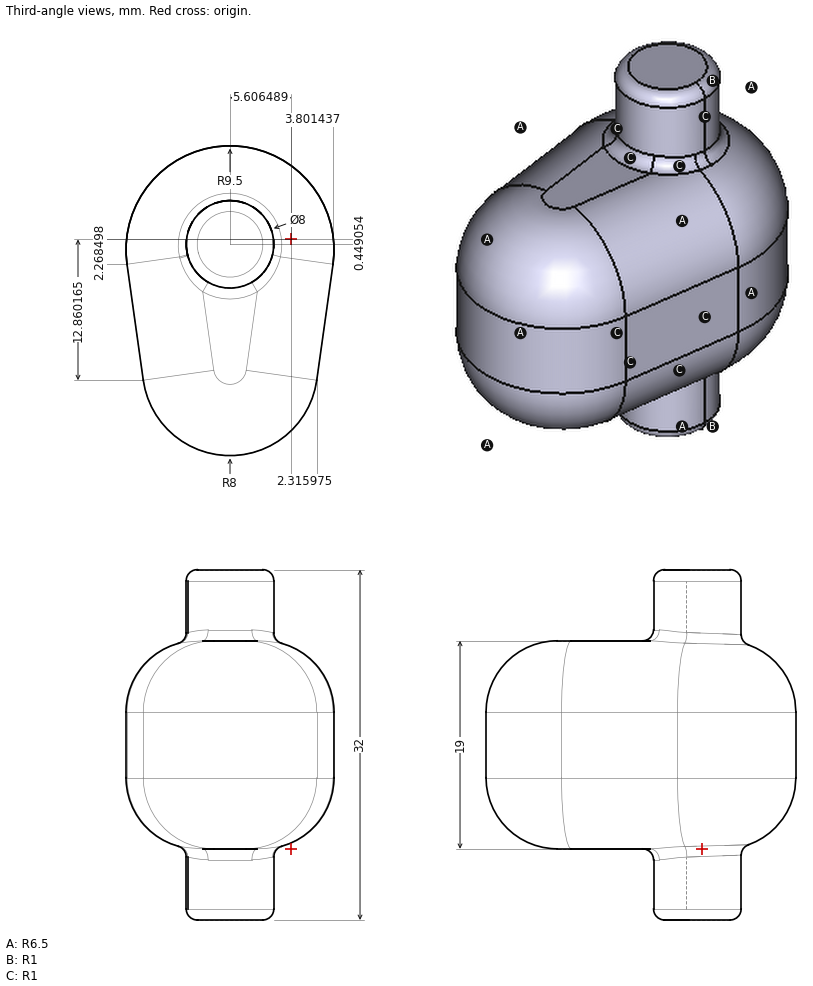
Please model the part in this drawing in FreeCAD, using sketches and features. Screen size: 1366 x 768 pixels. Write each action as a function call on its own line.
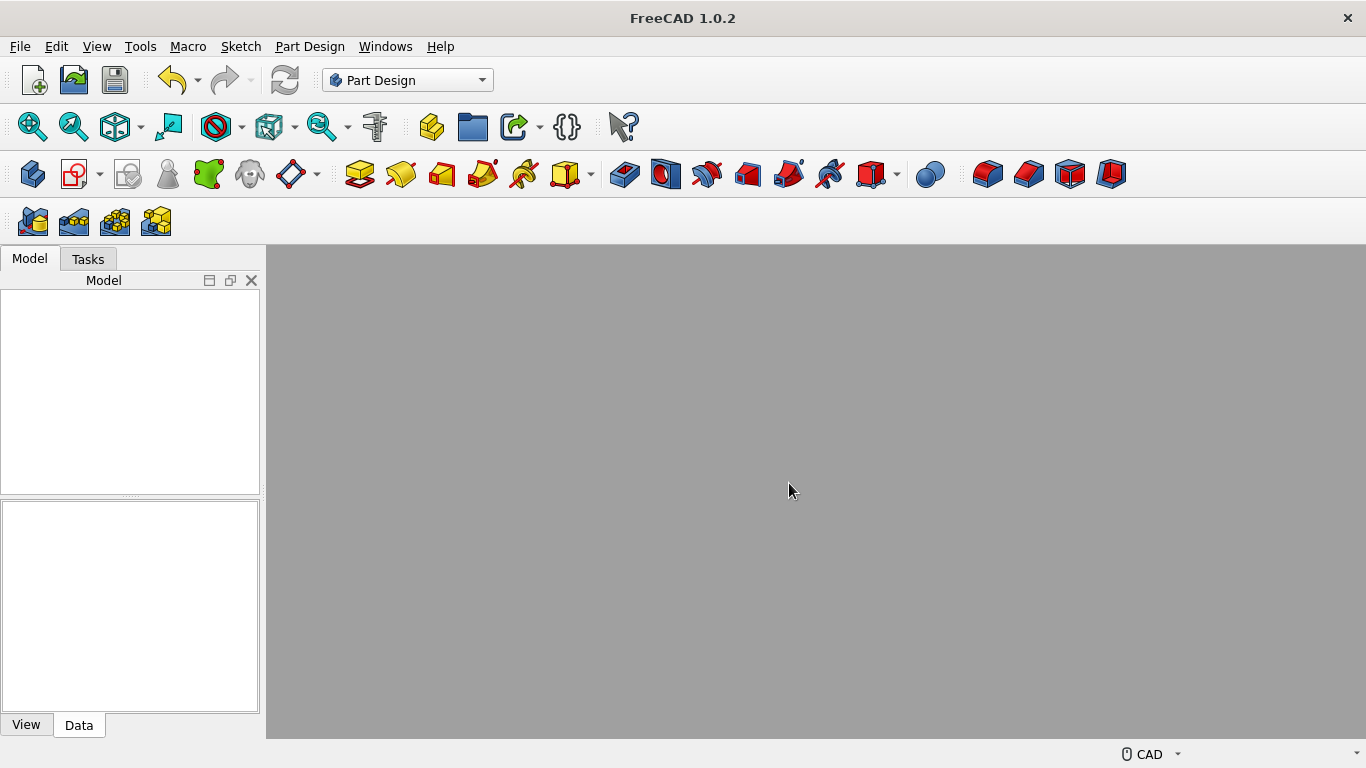
key(ctrl+n)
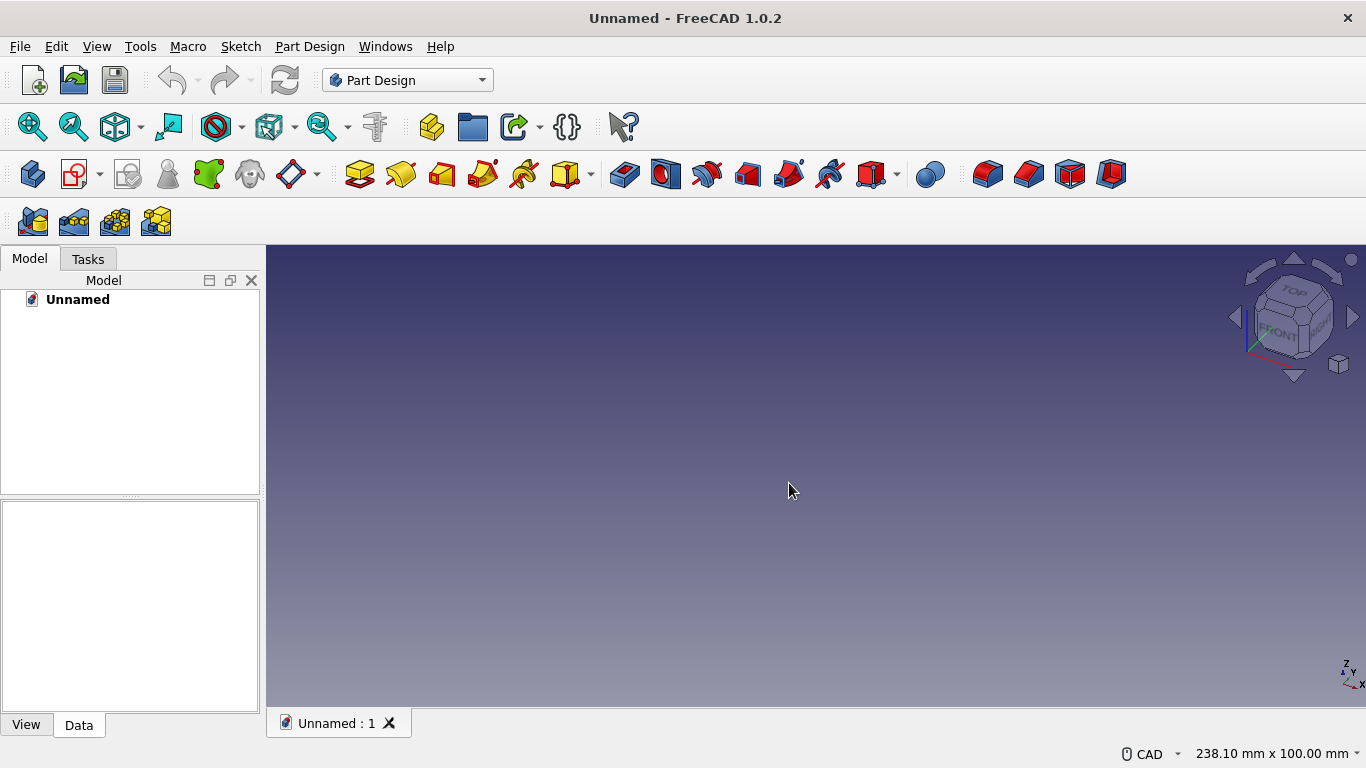
click(74, 174)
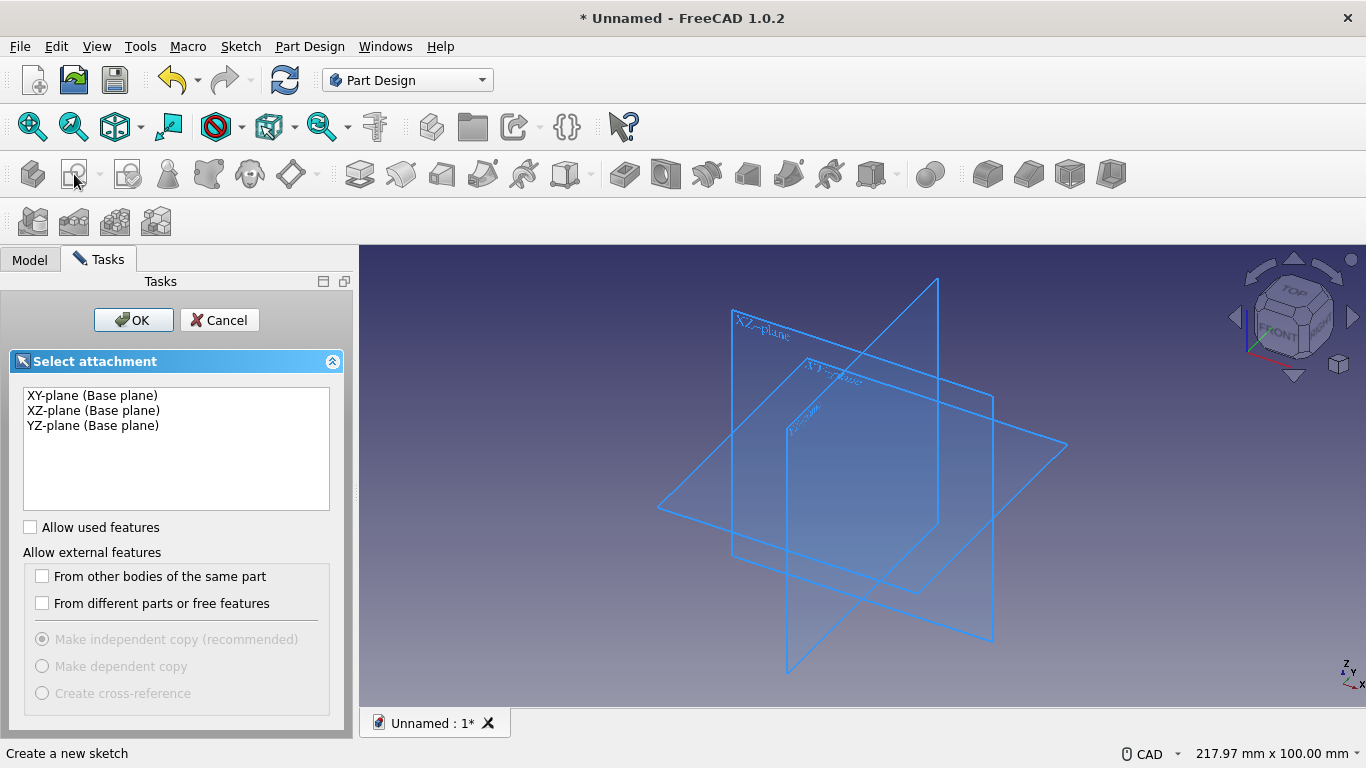
click(84, 396)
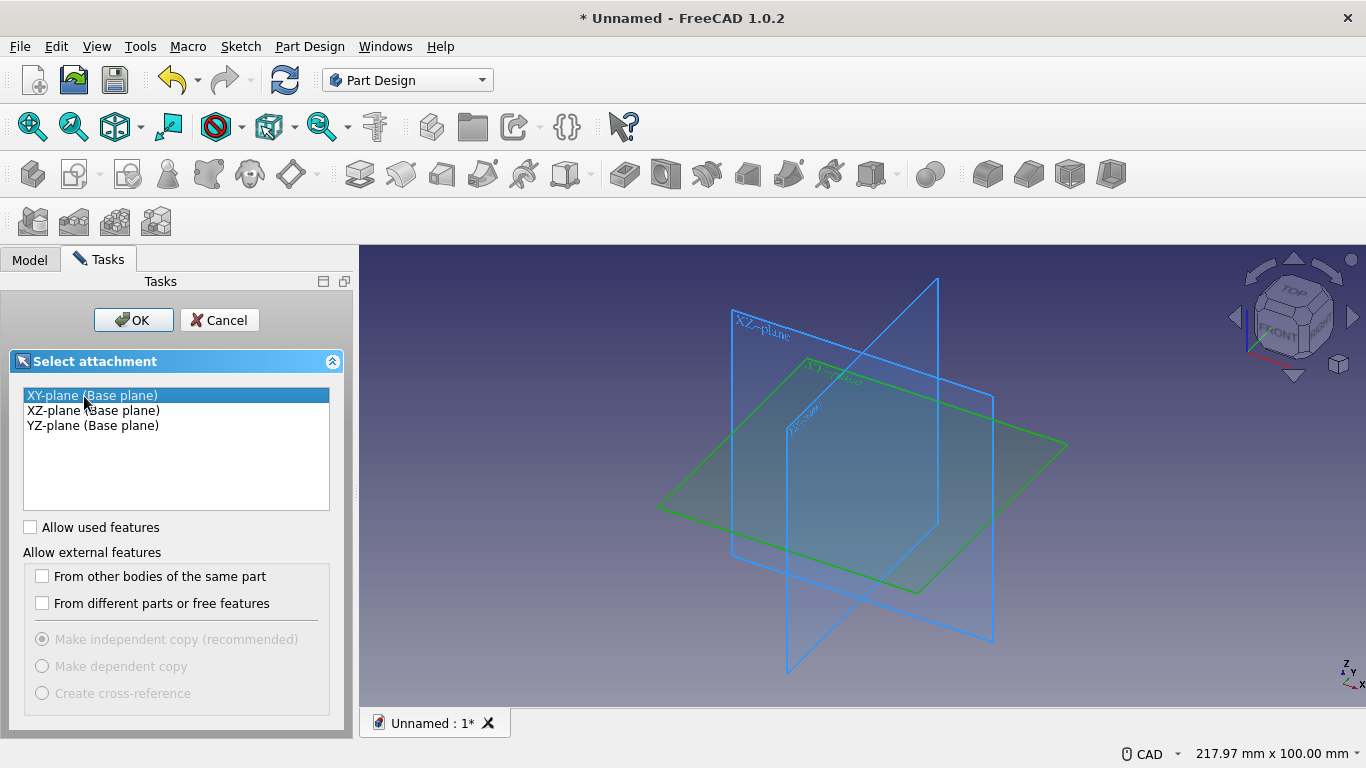
click(134, 320)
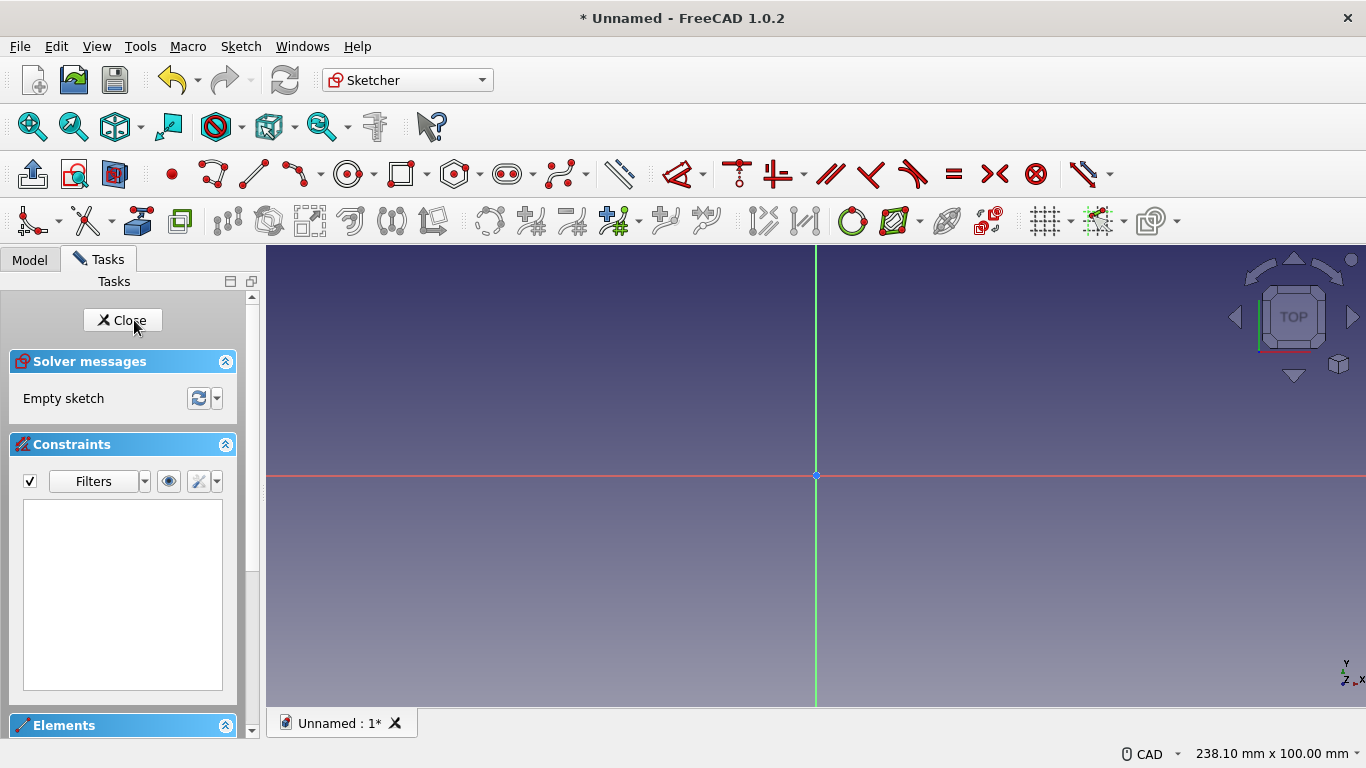
scroll(825, 523, up, 4)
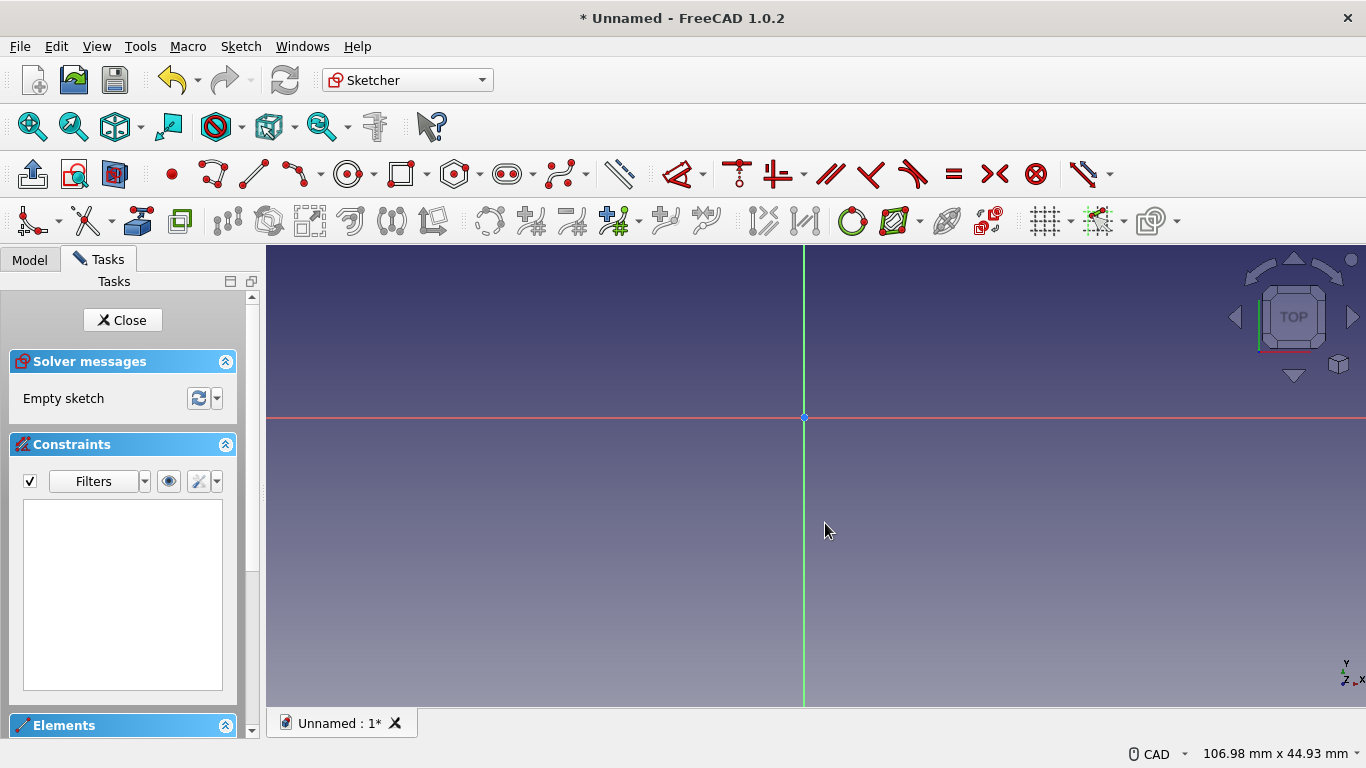
key(g)
key(l)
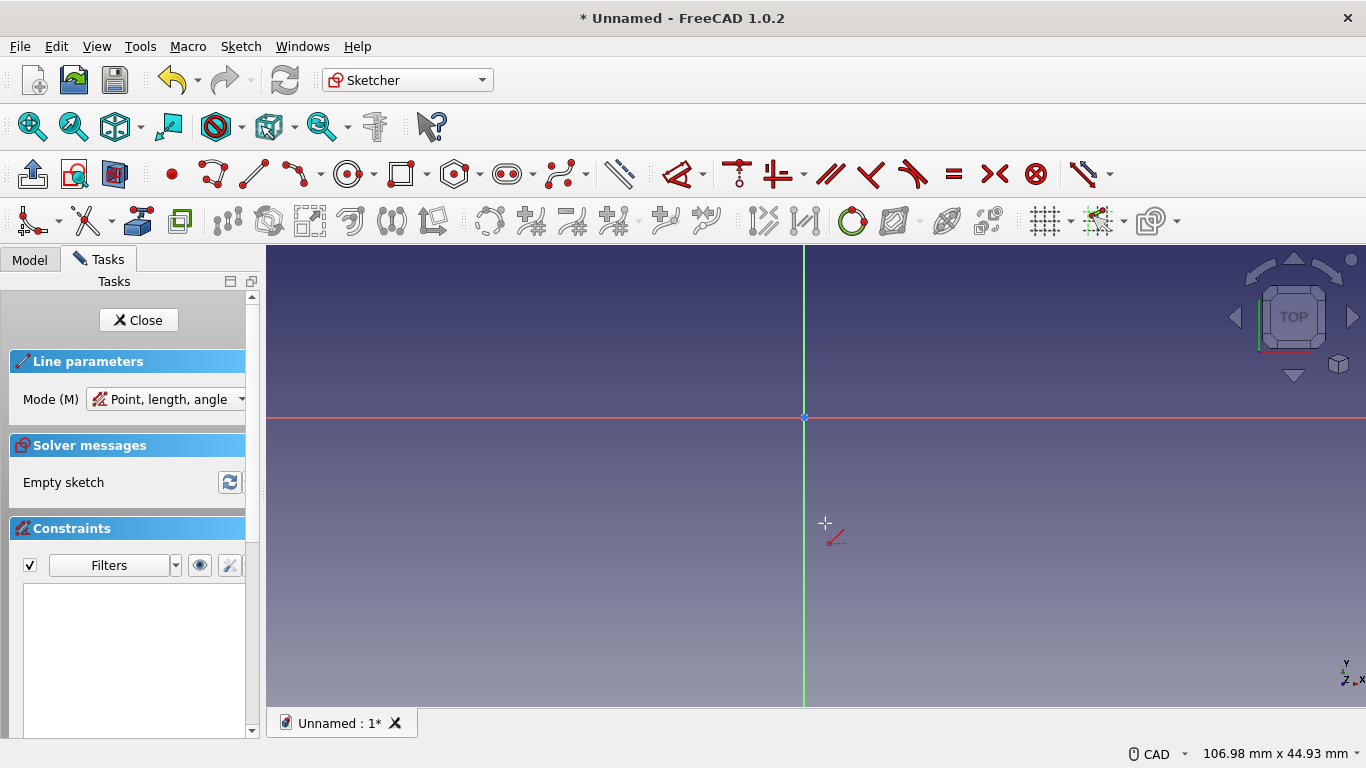
click(650, 441)
click(665, 550)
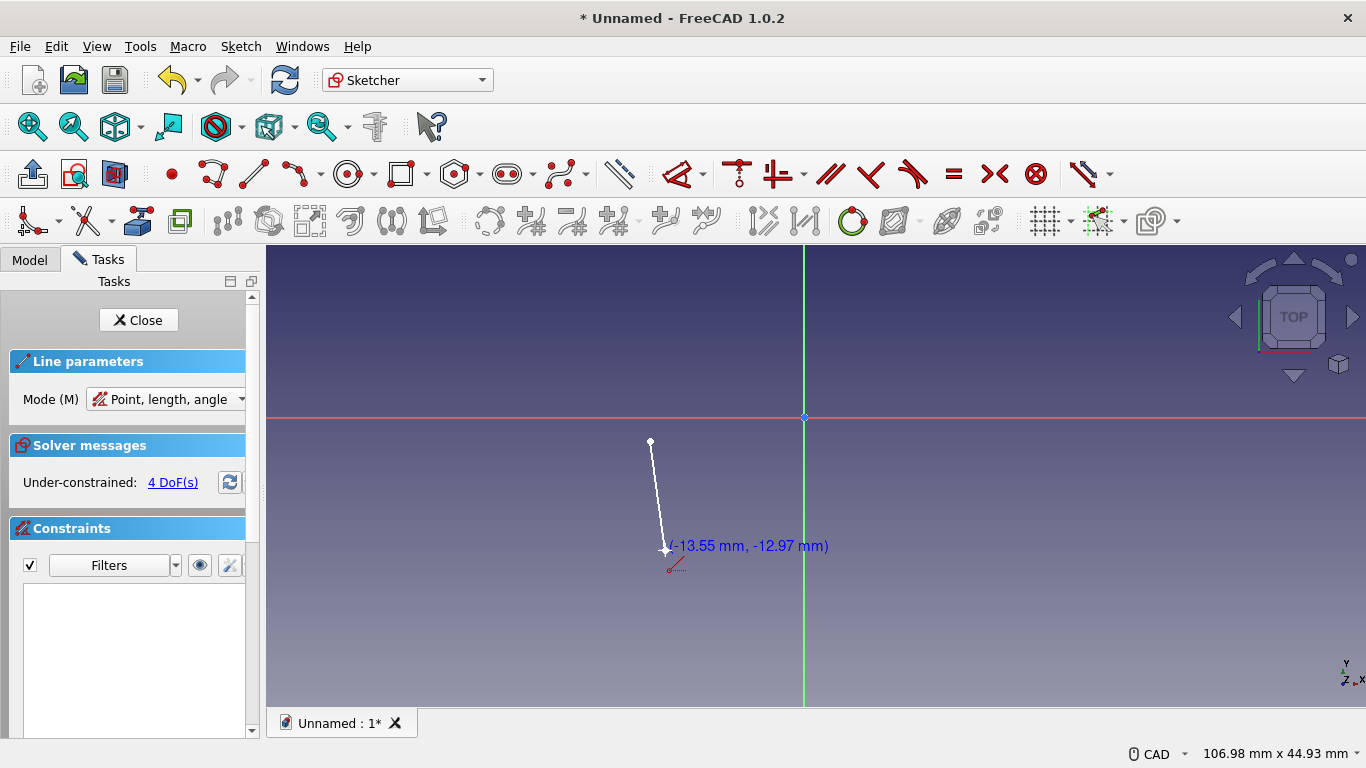
click(828, 550)
click(843, 441)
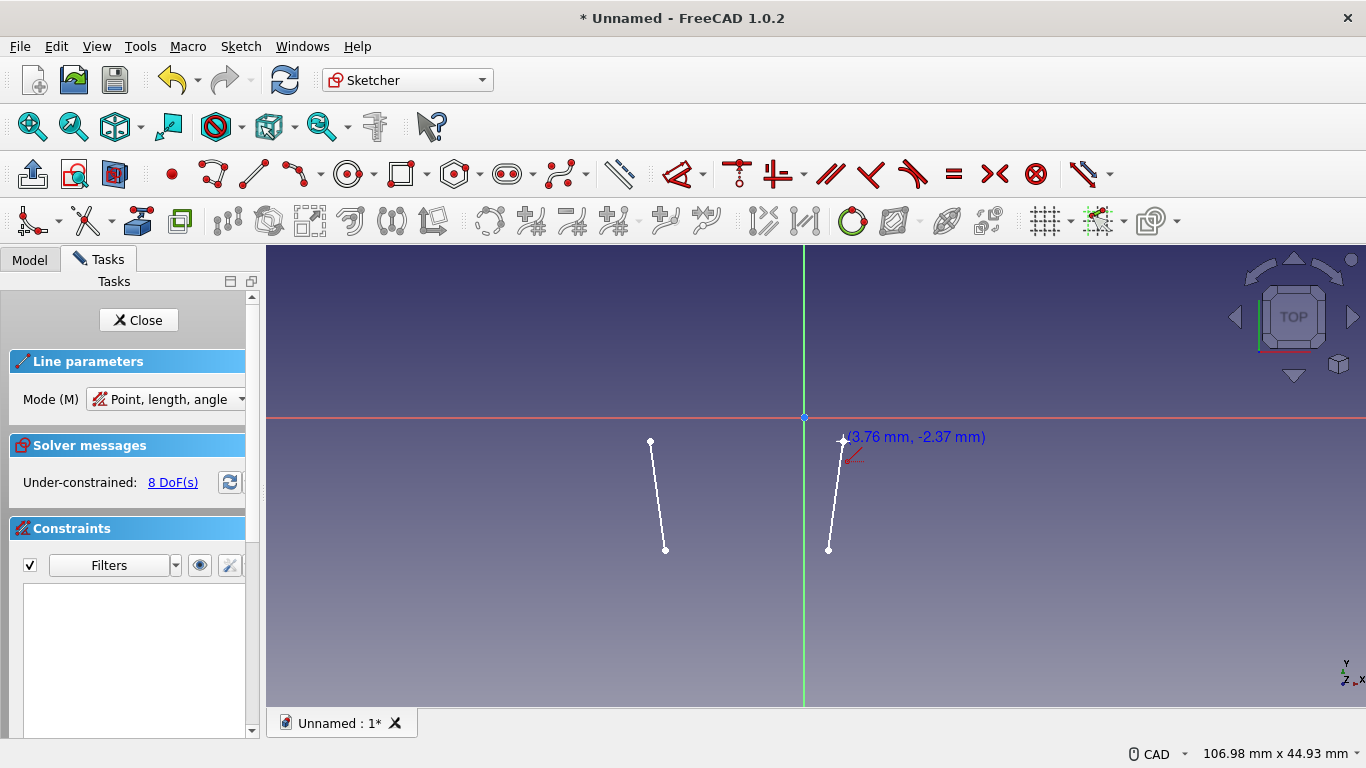
key(g)
key(3)
key(a)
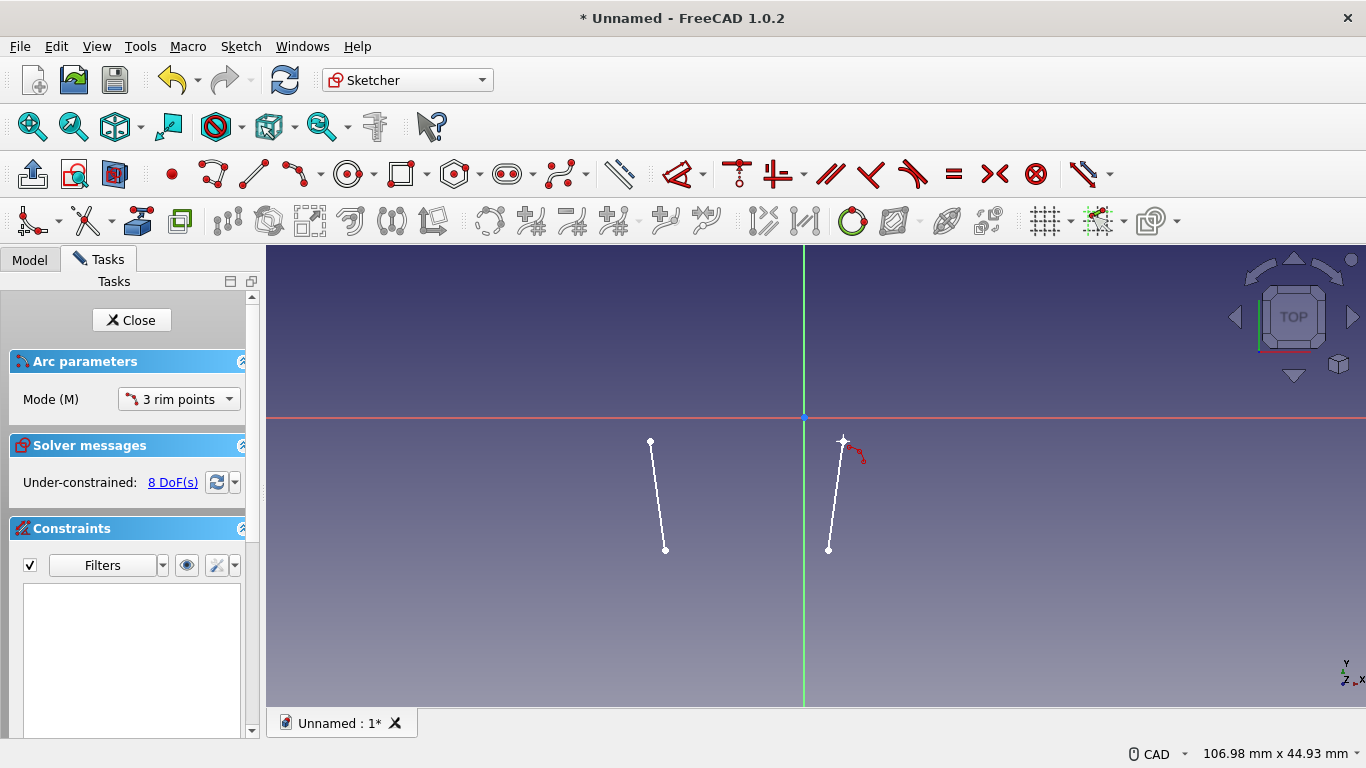
click(665, 551)
click(828, 551)
click(747, 621)